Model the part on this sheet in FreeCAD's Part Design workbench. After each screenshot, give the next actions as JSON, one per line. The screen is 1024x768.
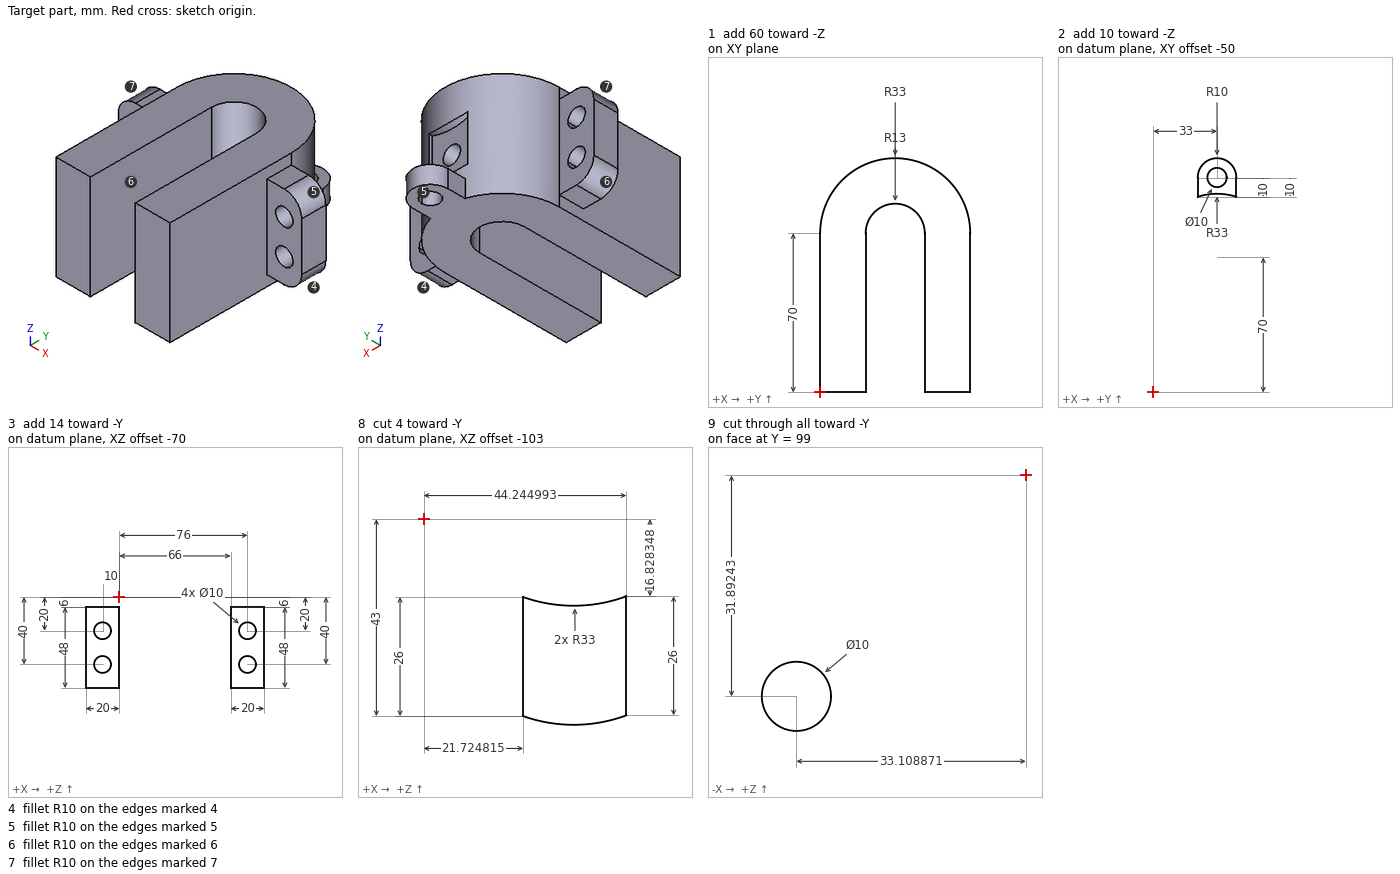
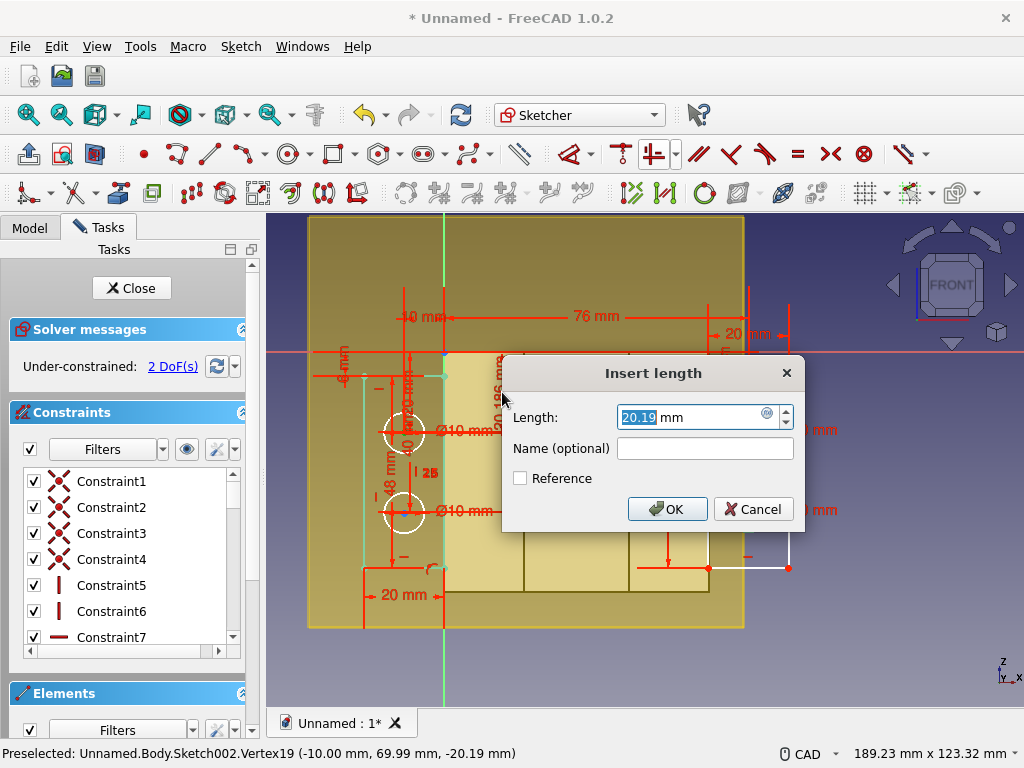
{"action": "type", "text": "20"}
{"action": "key", "text": "Return"}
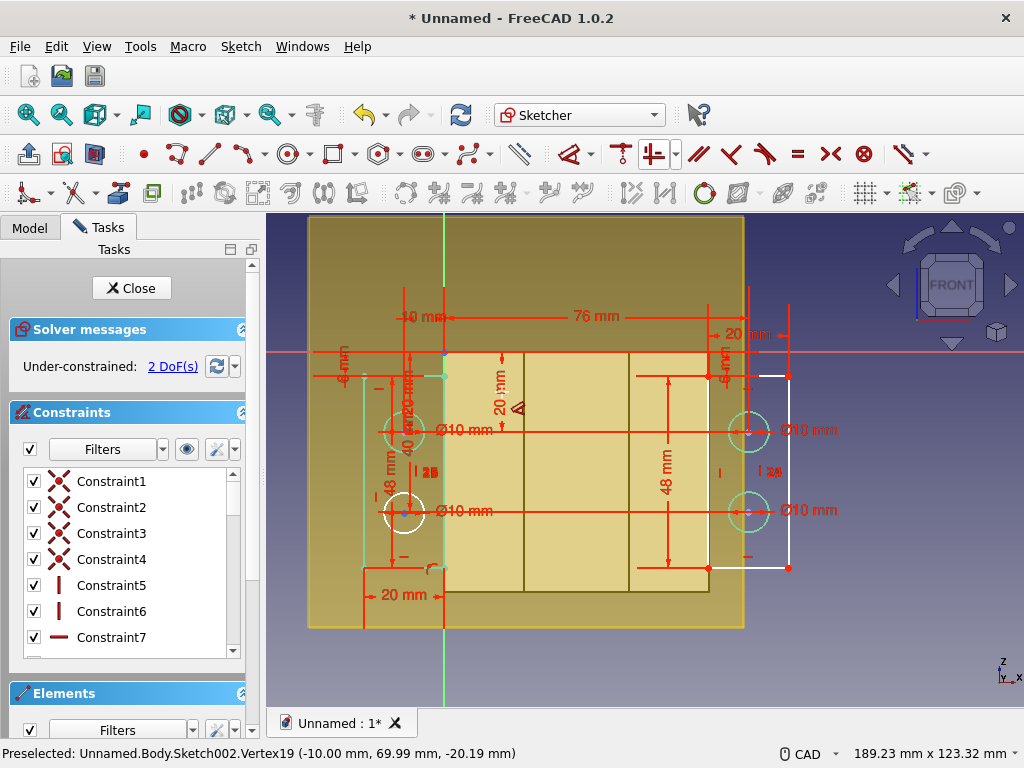
{"action": "left_click", "coordinate": [404, 513]}
{"action": "left_click", "coordinate": [478, 470]}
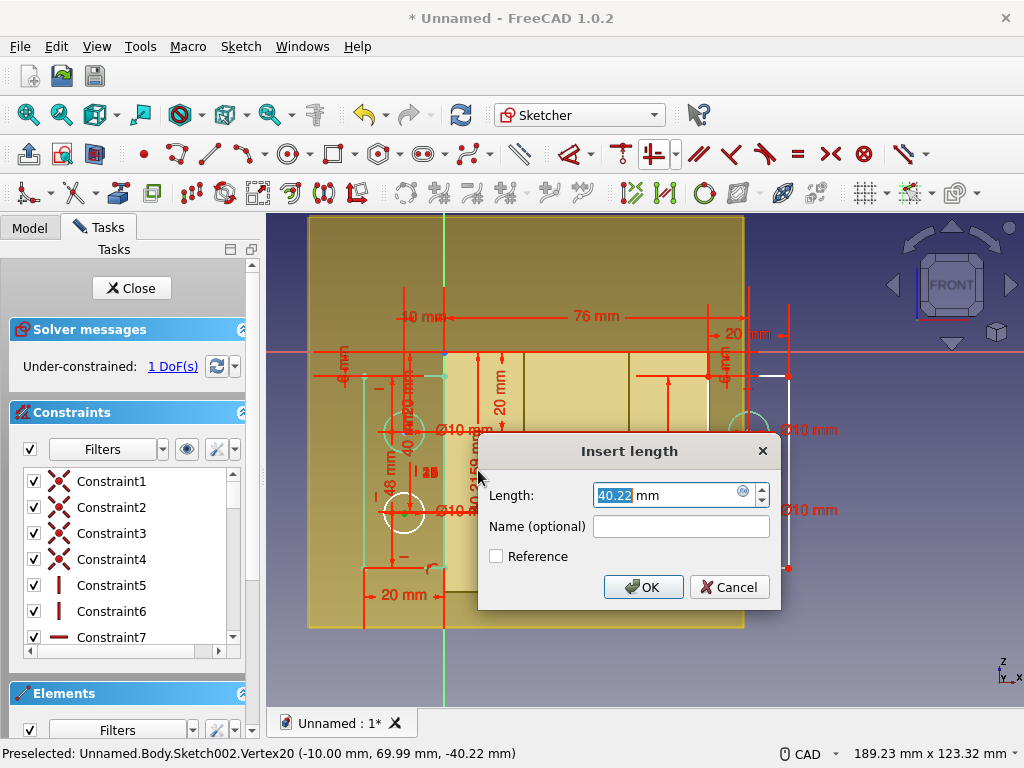
{"action": "type", "text": "40"}
{"action": "key", "text": "Return"}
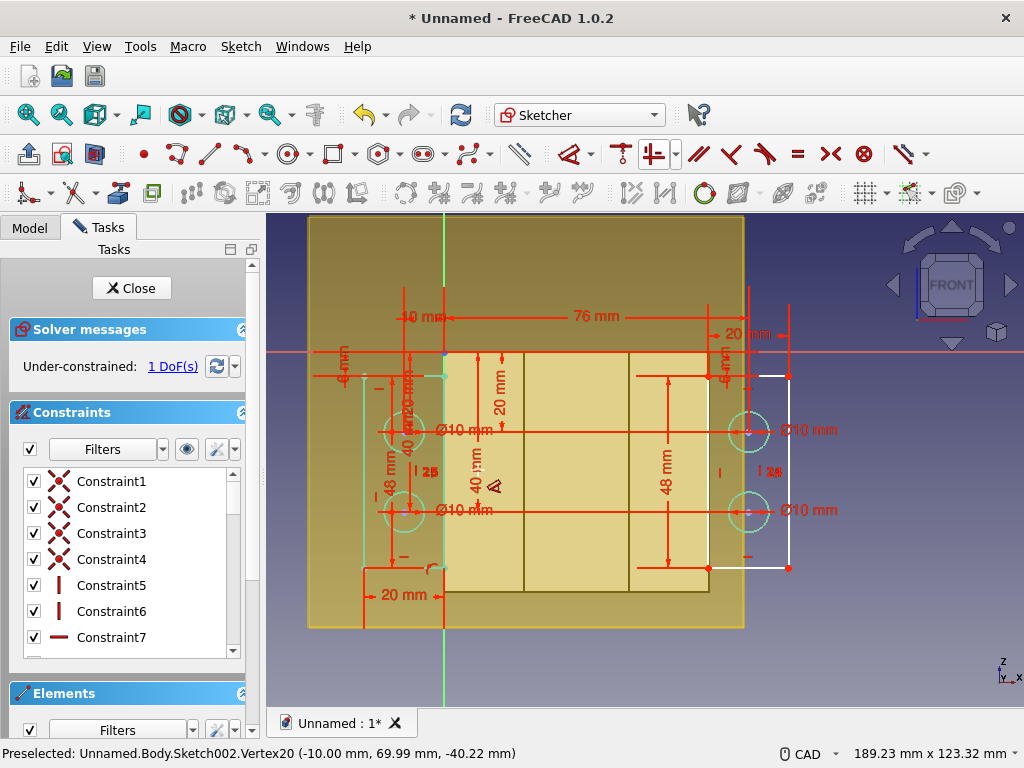
{"action": "left_click", "coordinate": [708, 376]}
{"action": "left_click", "coordinate": [516, 318]}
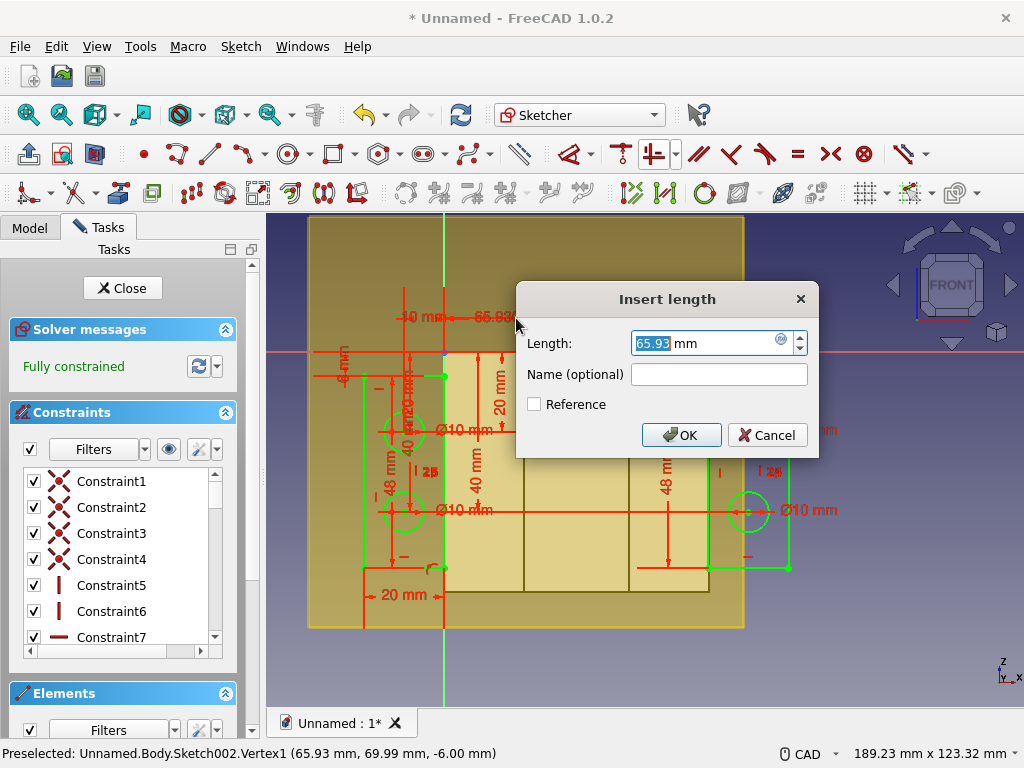
{"action": "type", "text": "66"}
{"action": "key", "text": "Return"}
{"action": "key", "text": "Escape"}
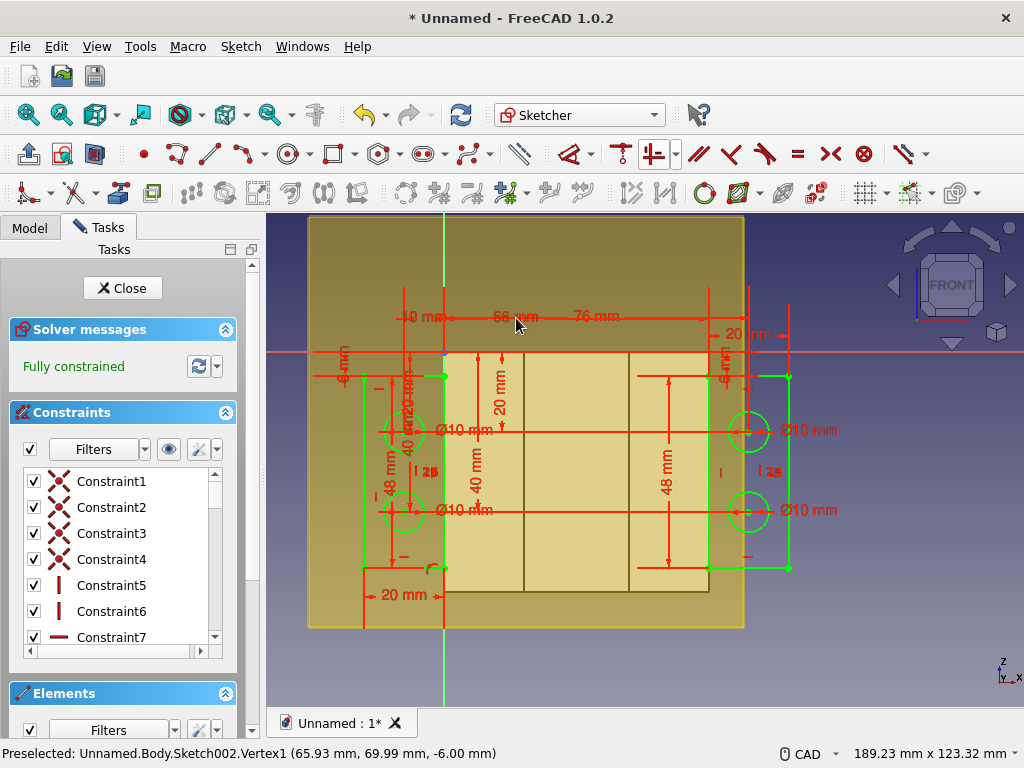
{"action": "left_click", "coordinate": [123, 288]}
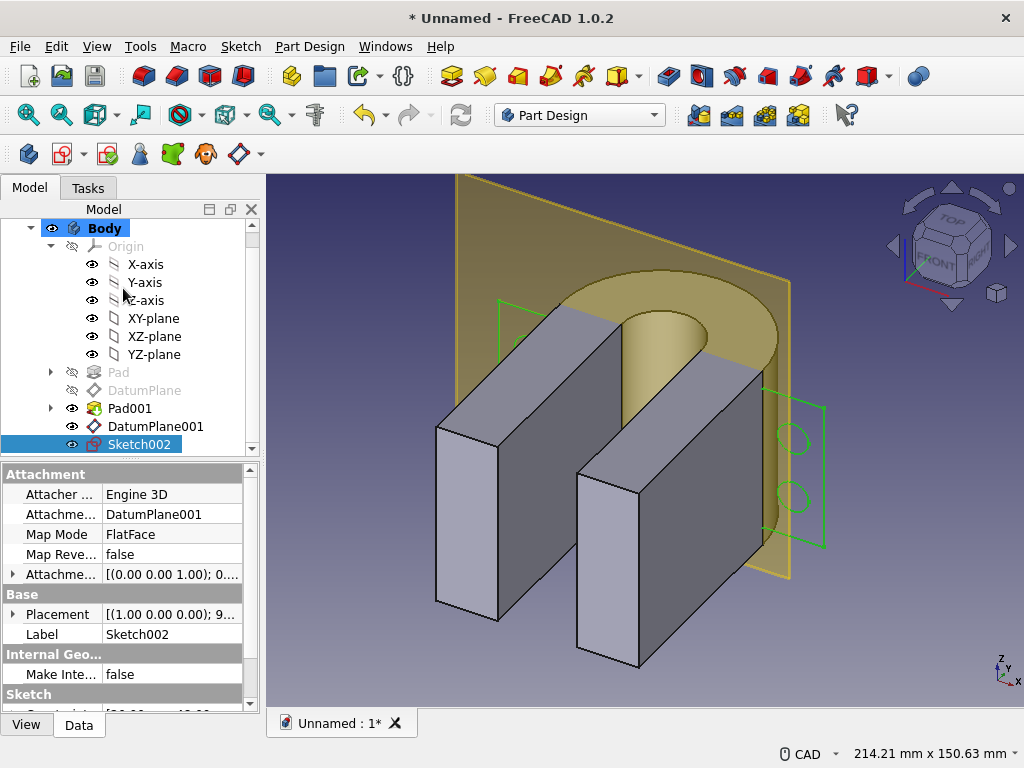
{"action": "left_click", "coordinate": [452, 76]}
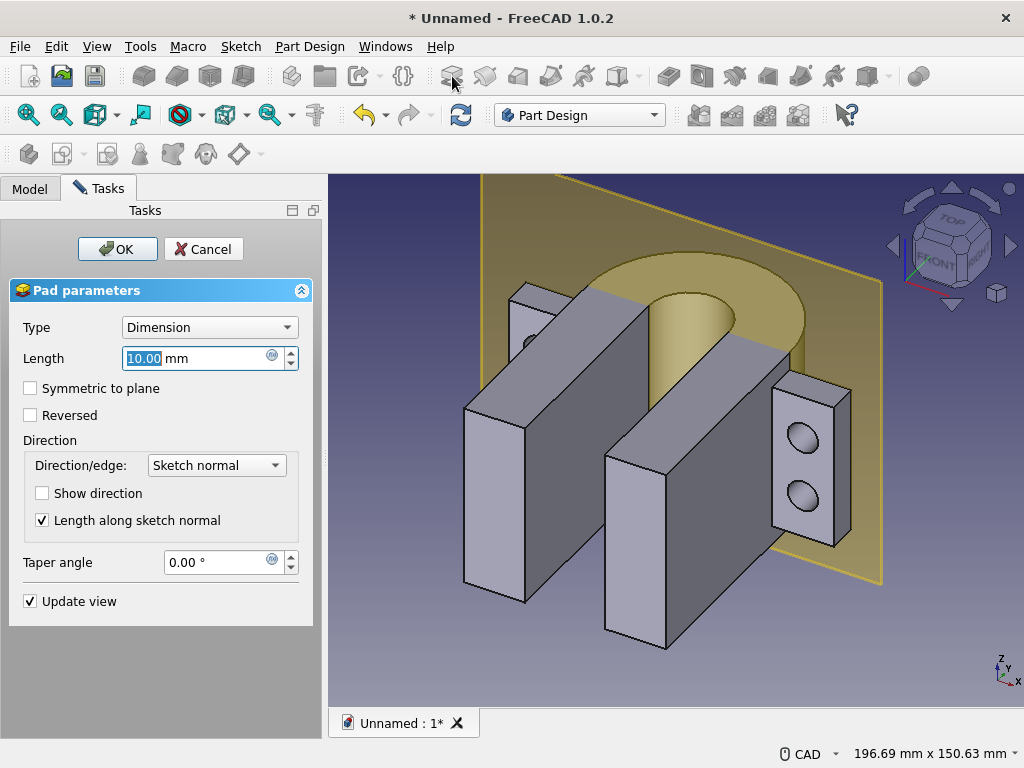
{"action": "type", "text": "14"}
{"action": "key", "text": "Tab"}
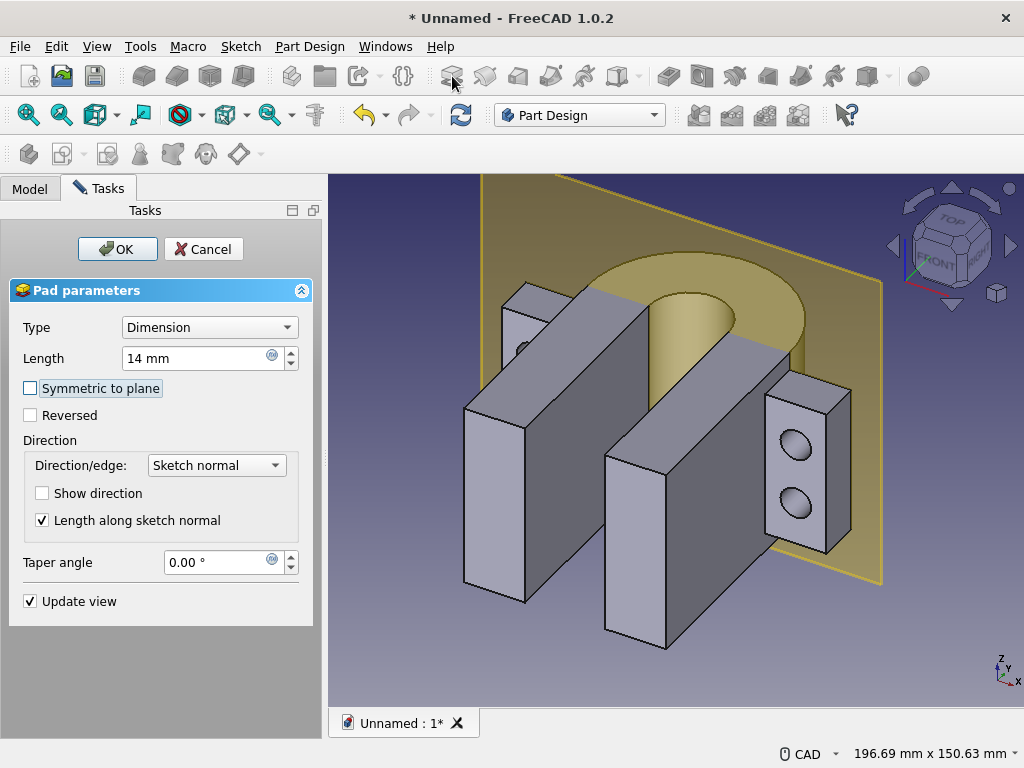
{"action": "left_click", "coordinate": [118, 249]}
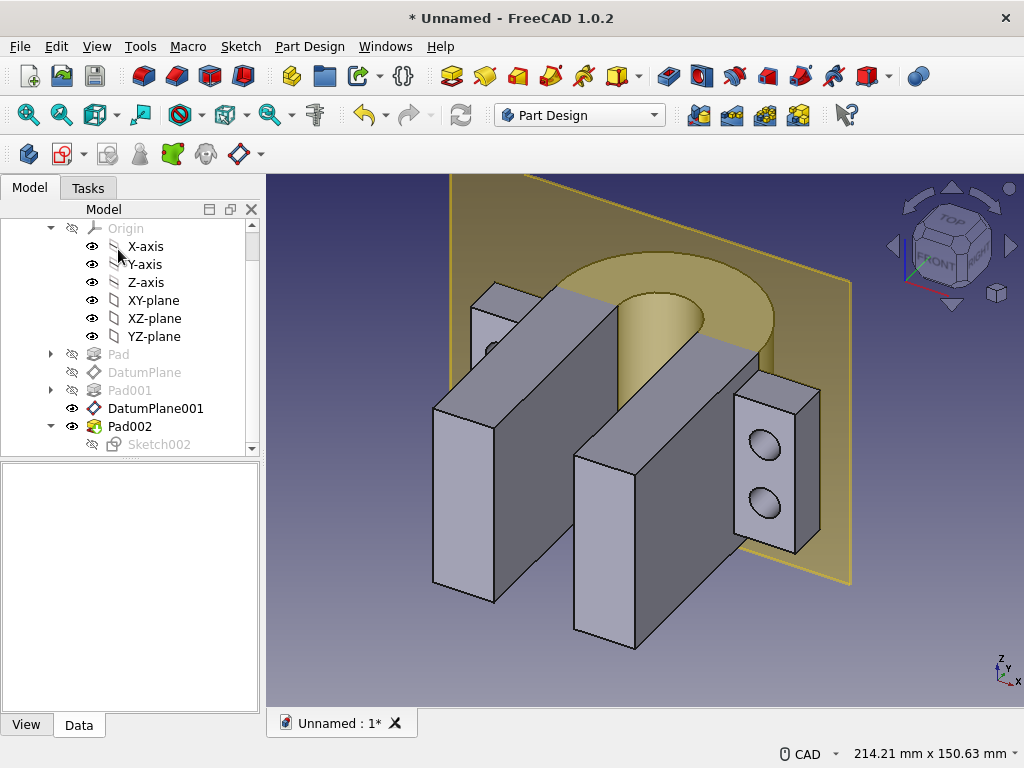
{"action": "left_click", "coordinate": [117, 408]}
{"action": "key", "text": "space"}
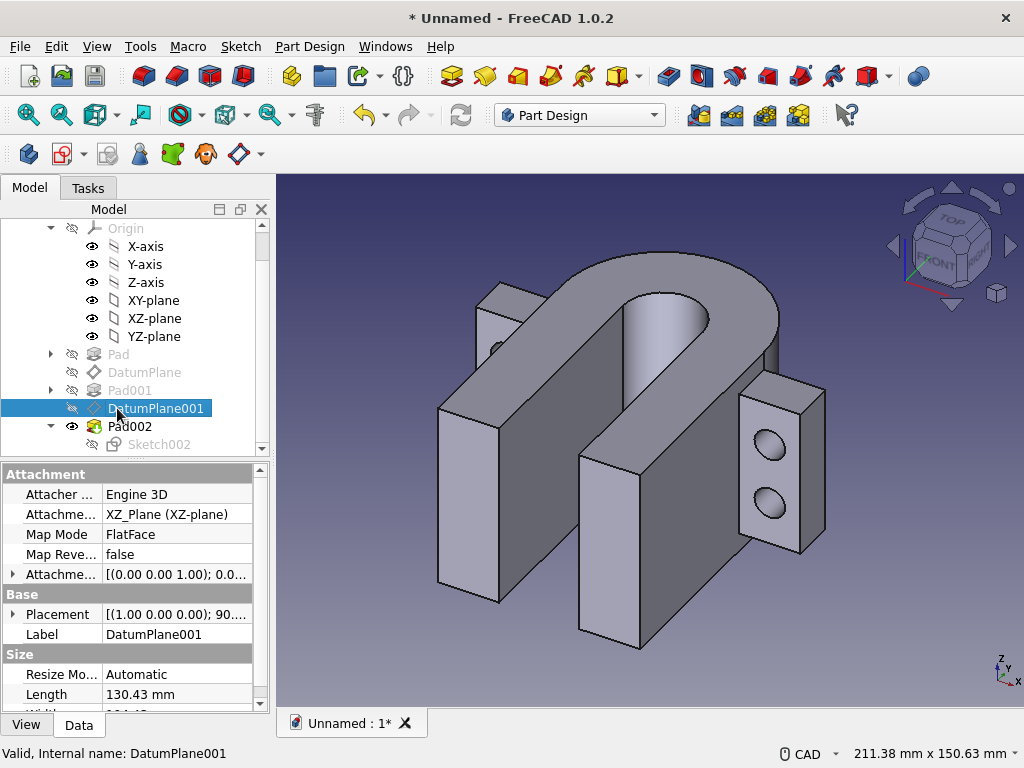
{"action": "key", "text": "0"}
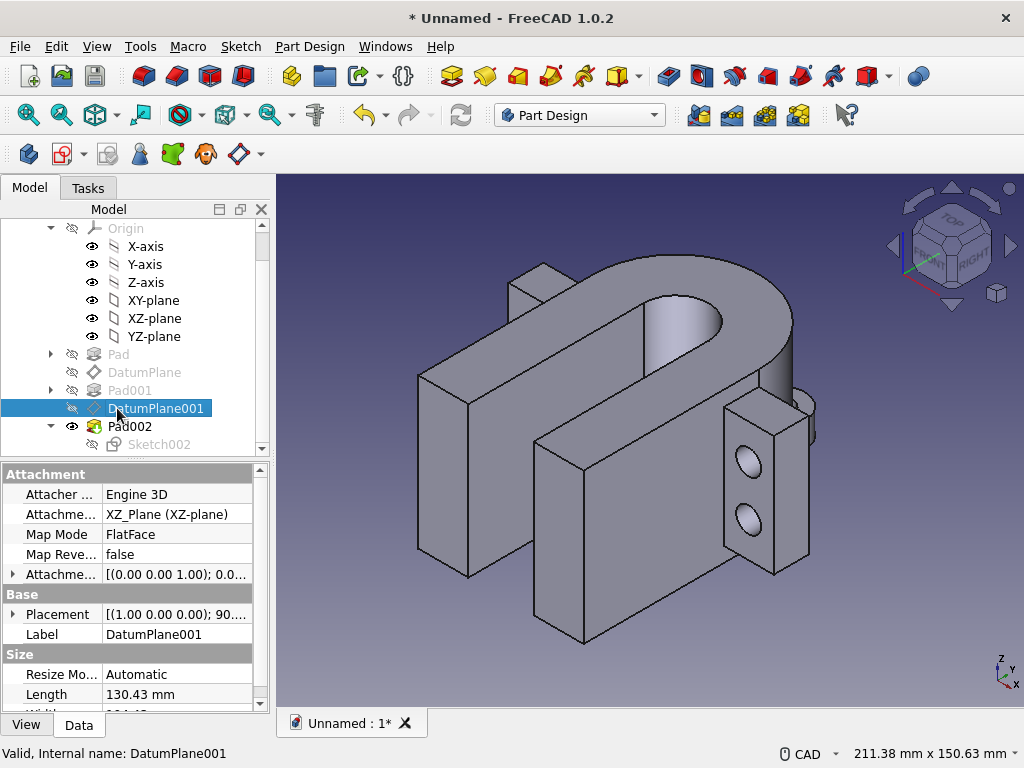
{"action": "left_click", "coordinate": [29, 116]}